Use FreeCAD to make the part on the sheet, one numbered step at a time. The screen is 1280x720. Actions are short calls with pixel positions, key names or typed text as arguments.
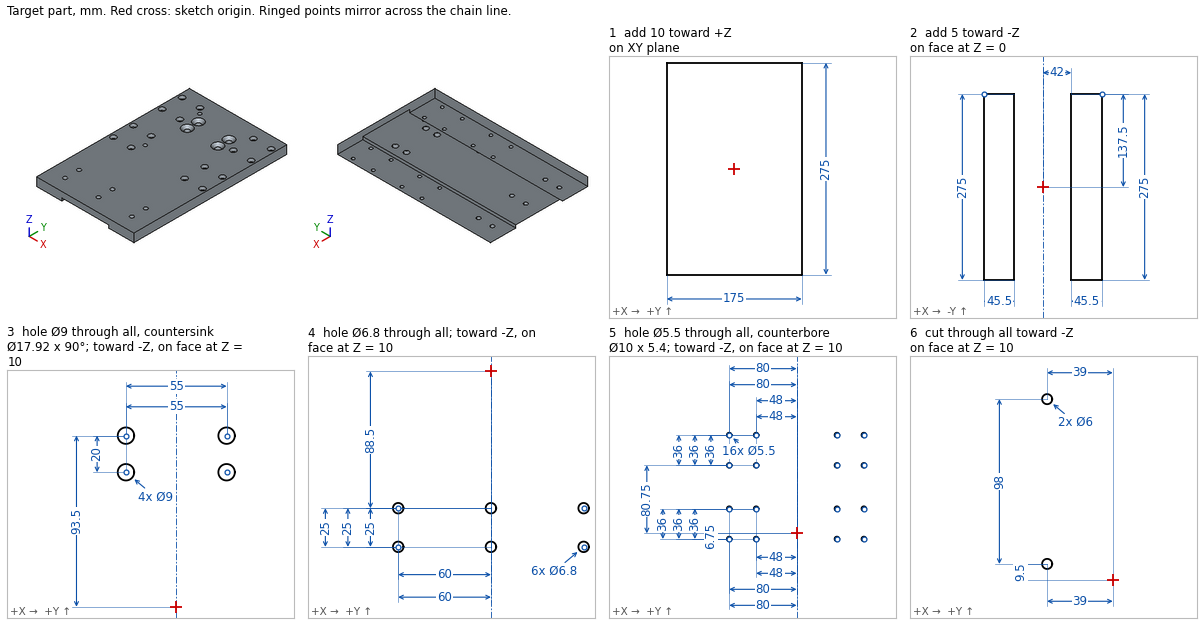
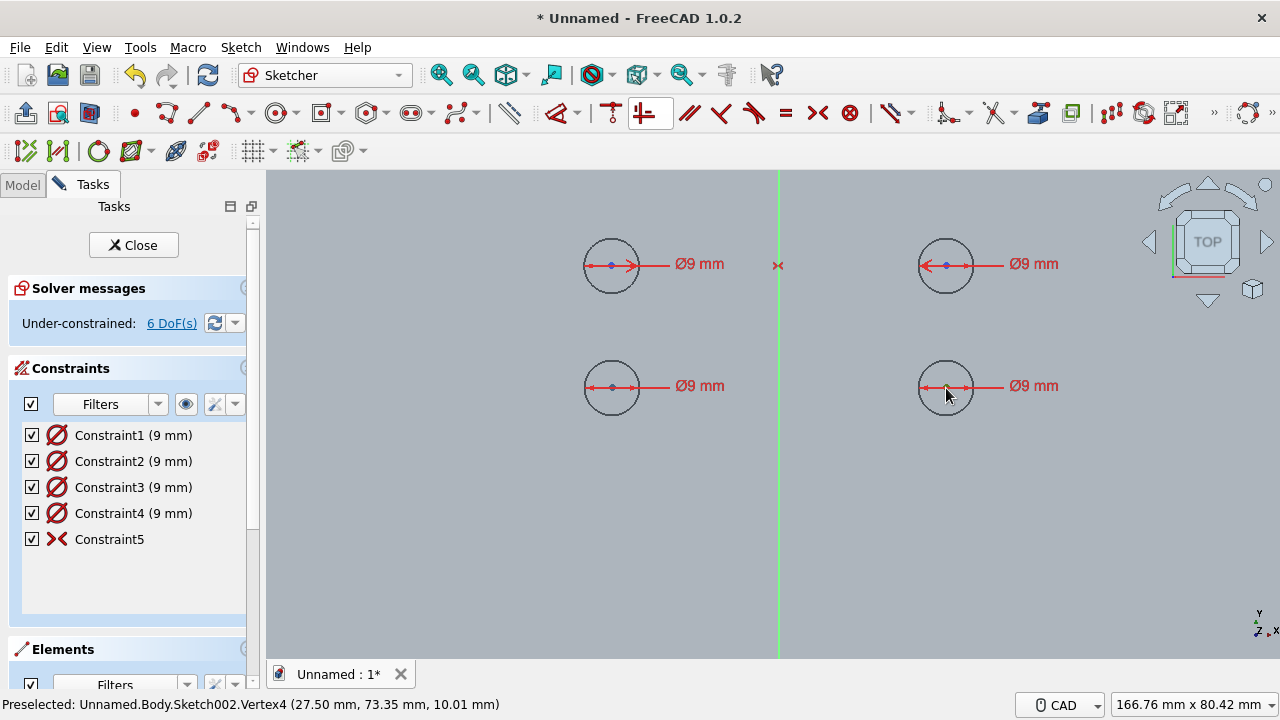
click(779, 600)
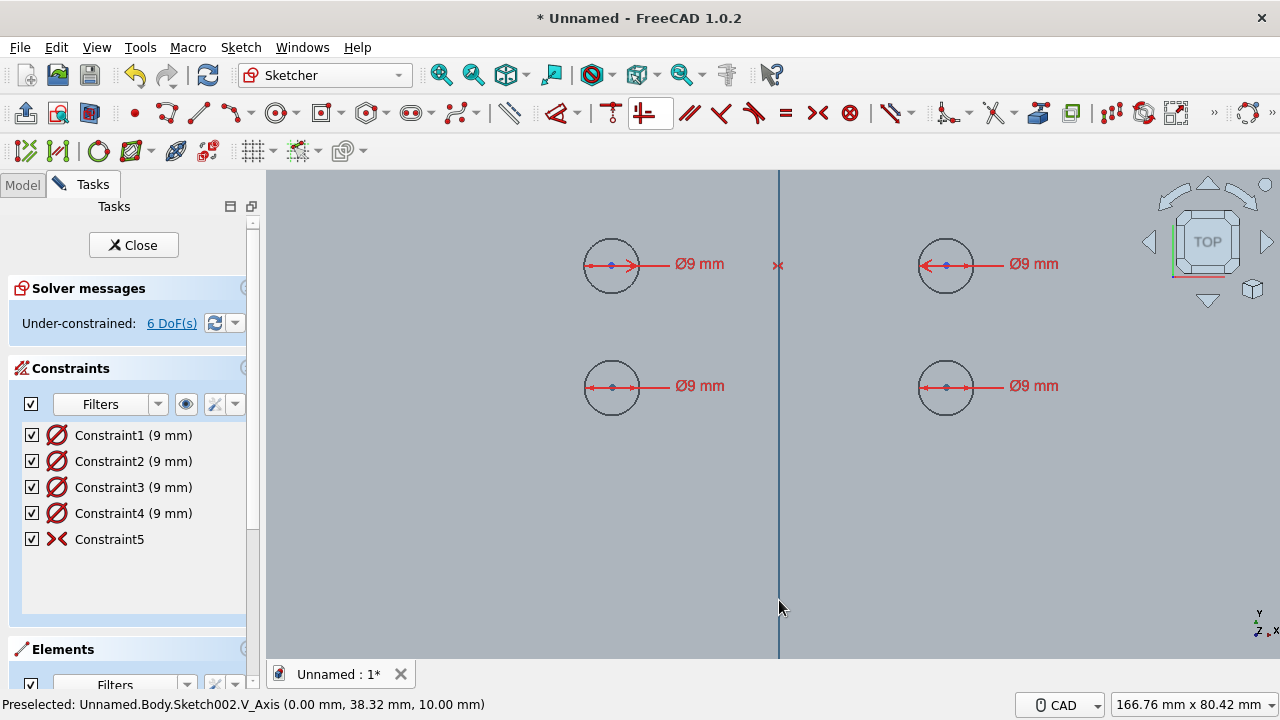
key(s)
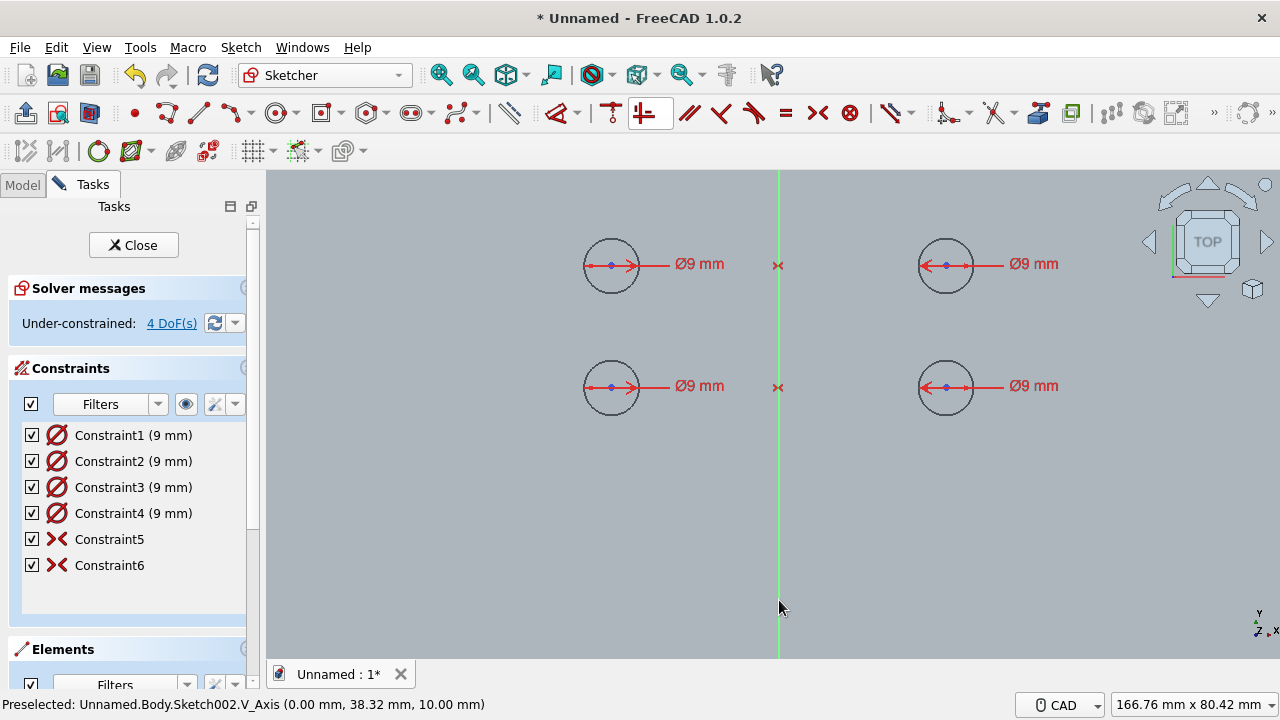
key(d)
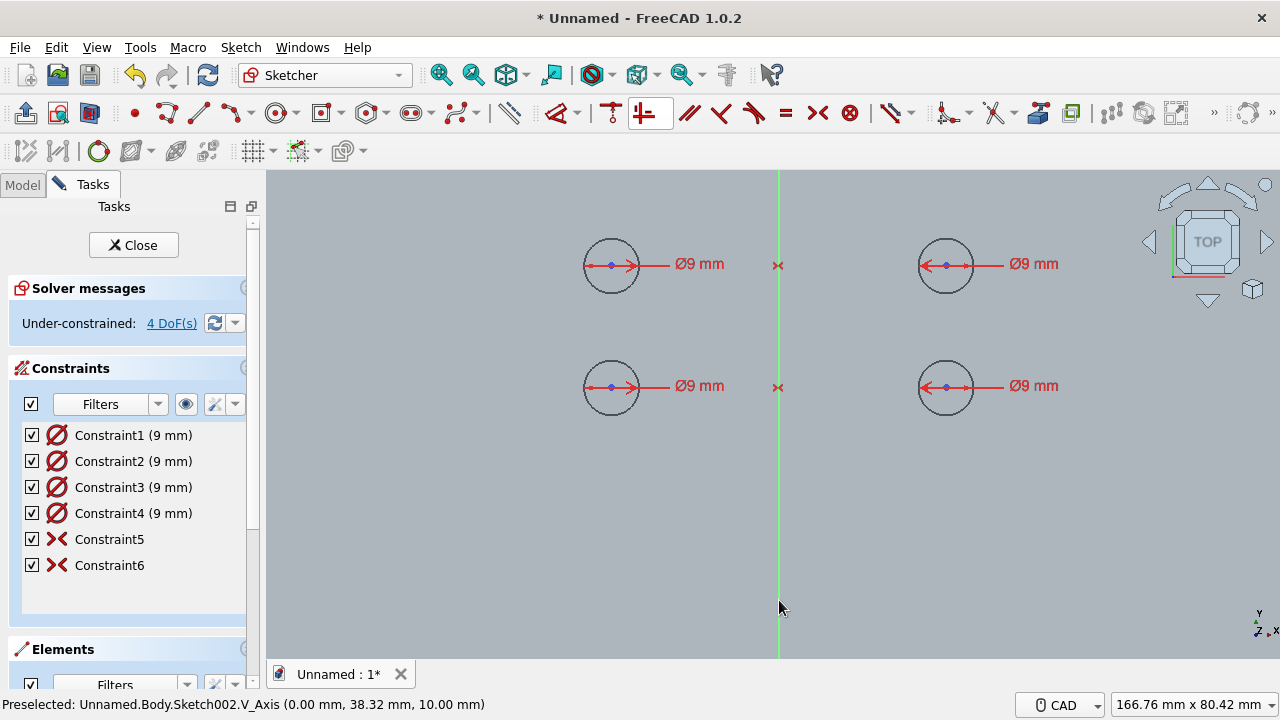
click(612, 266)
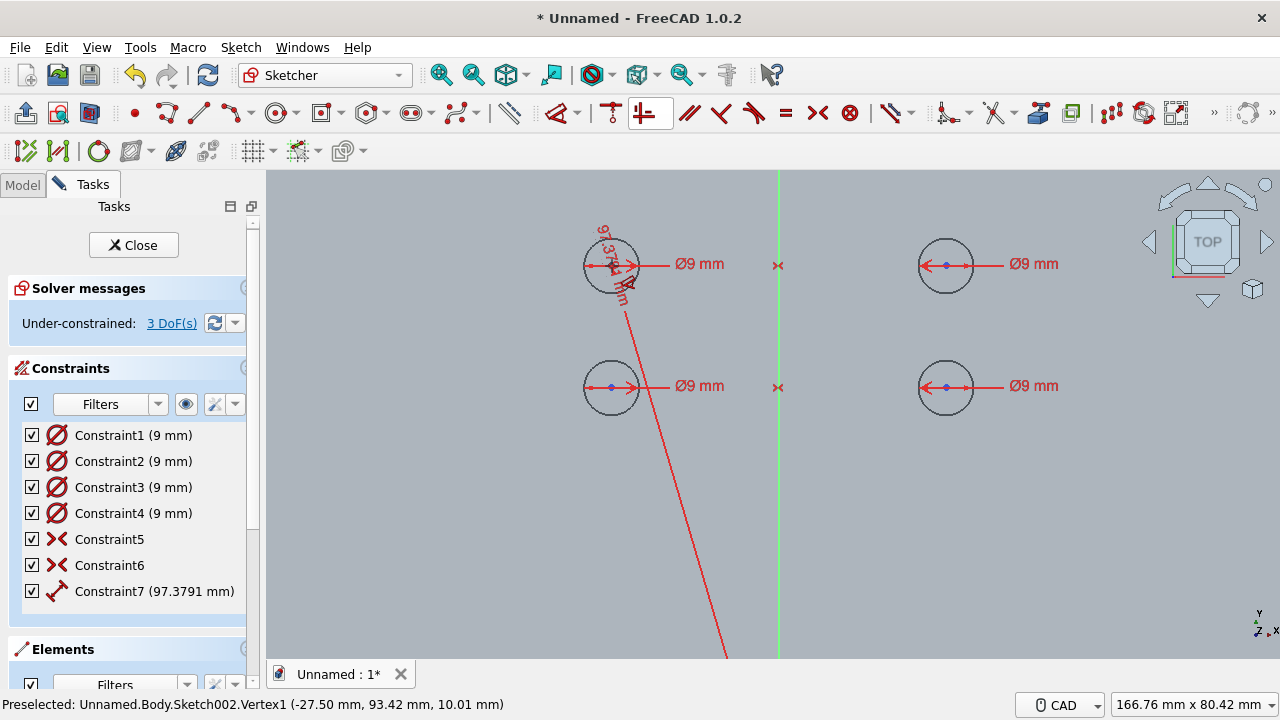
click(612, 388)
click(578, 327)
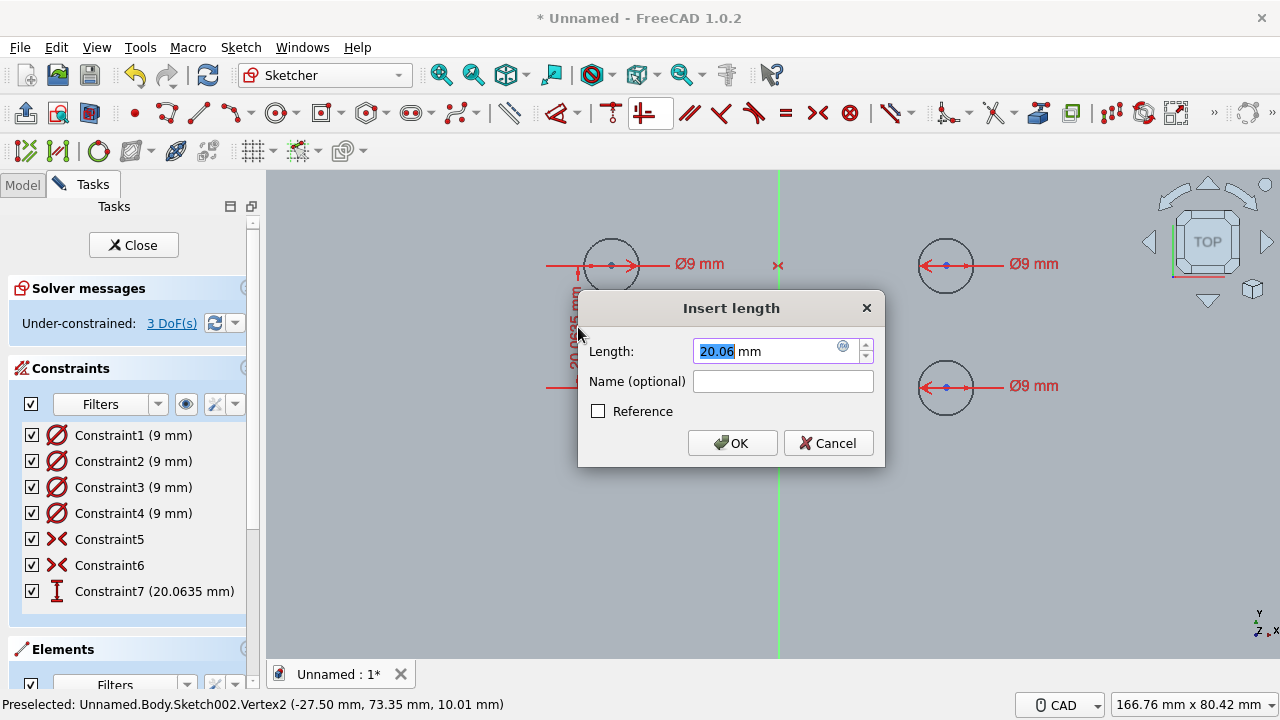
text(20)
key(Return)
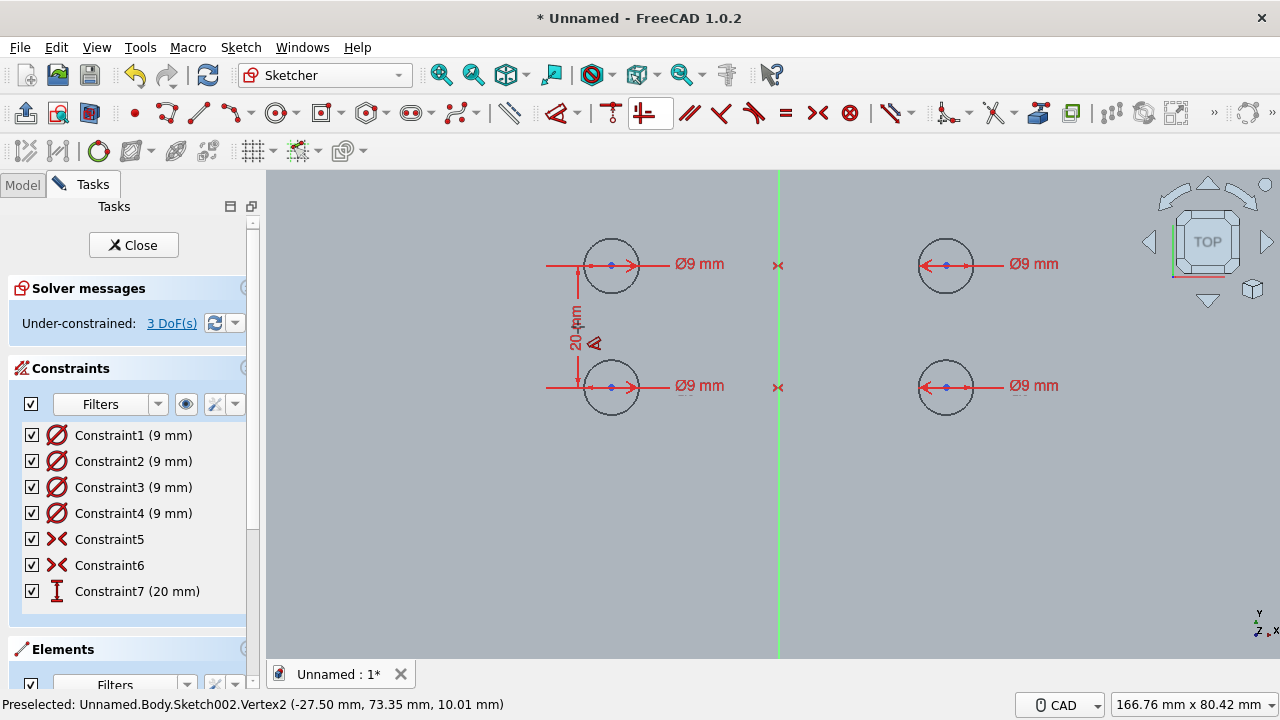
click(612, 266)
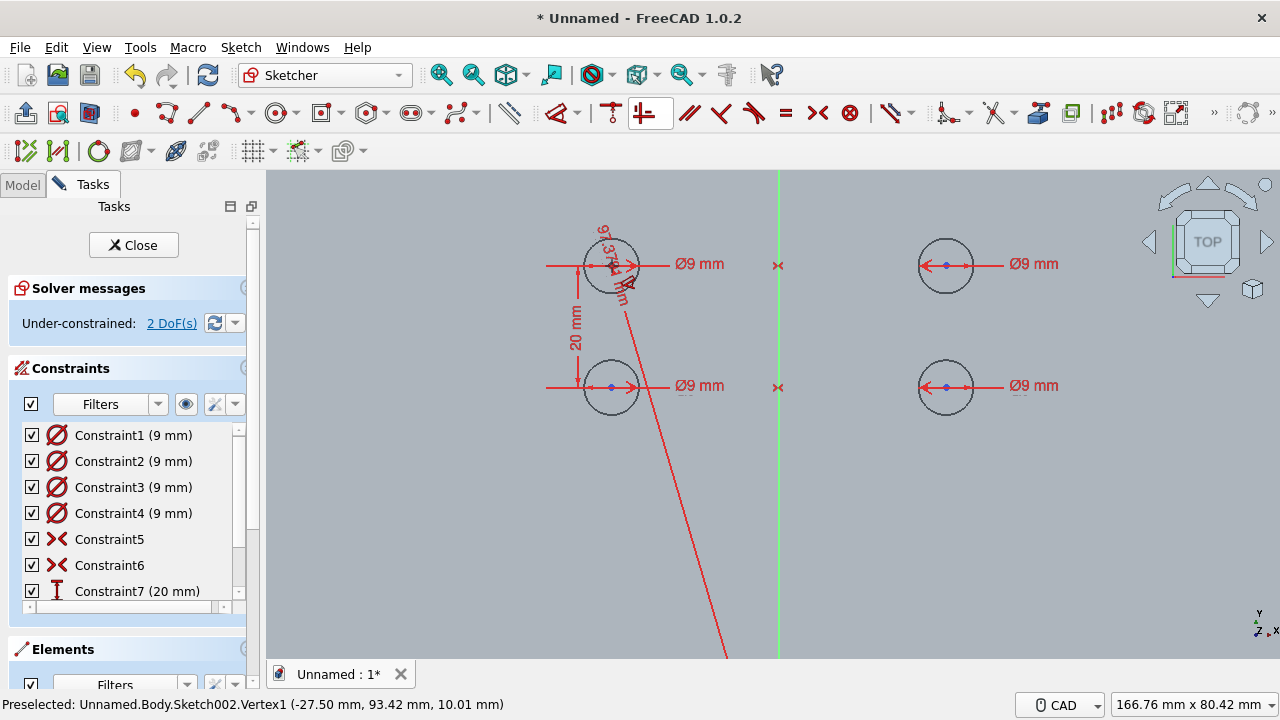
click(946, 266)
click(702, 232)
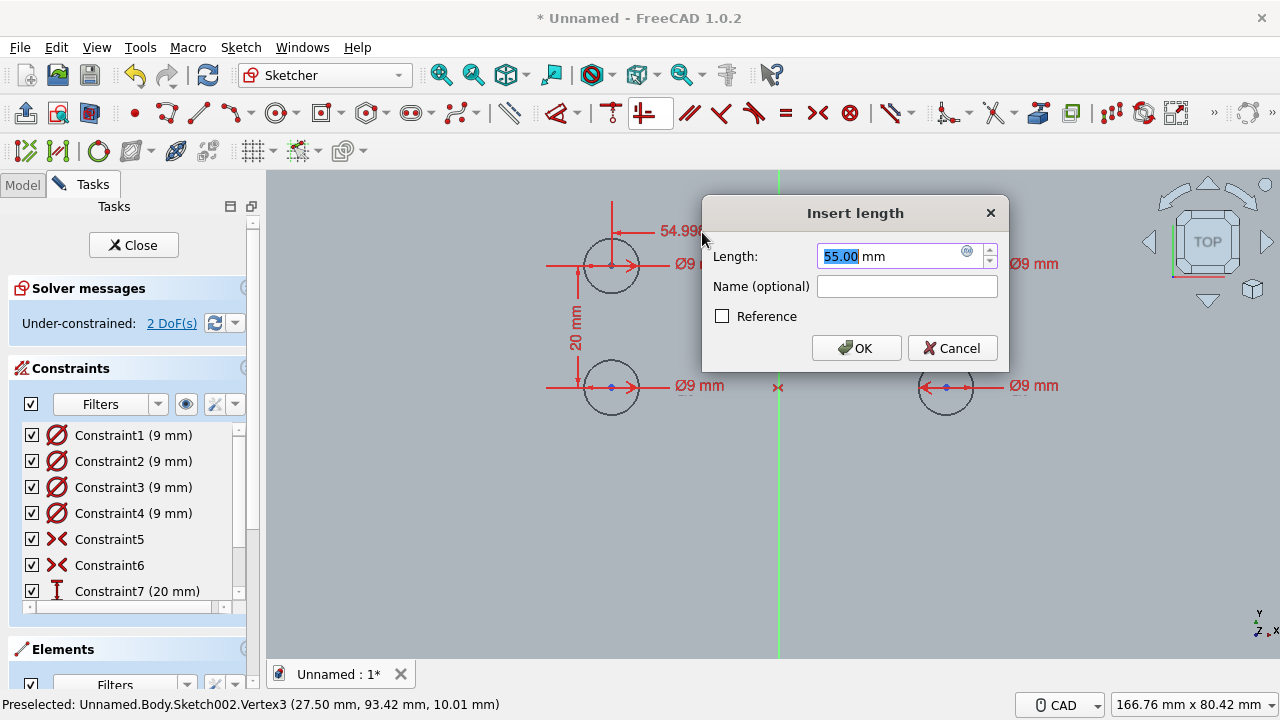
text(55)
key(Return)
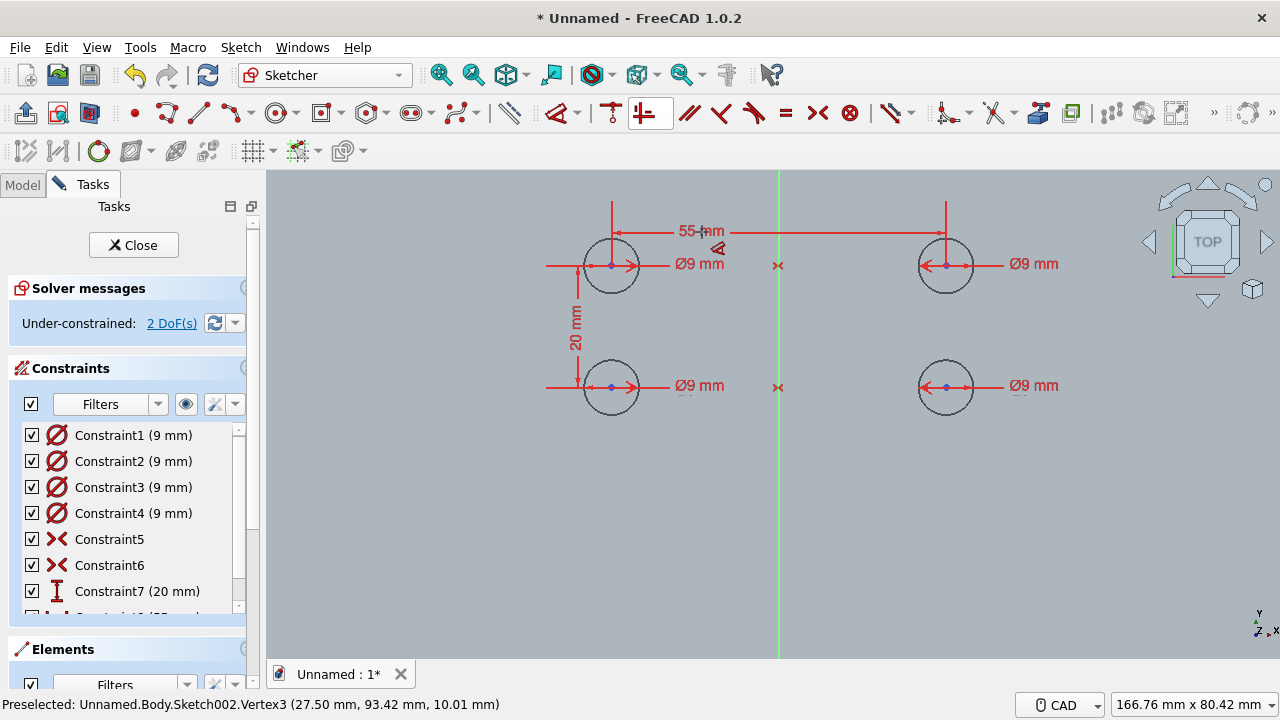
click(612, 388)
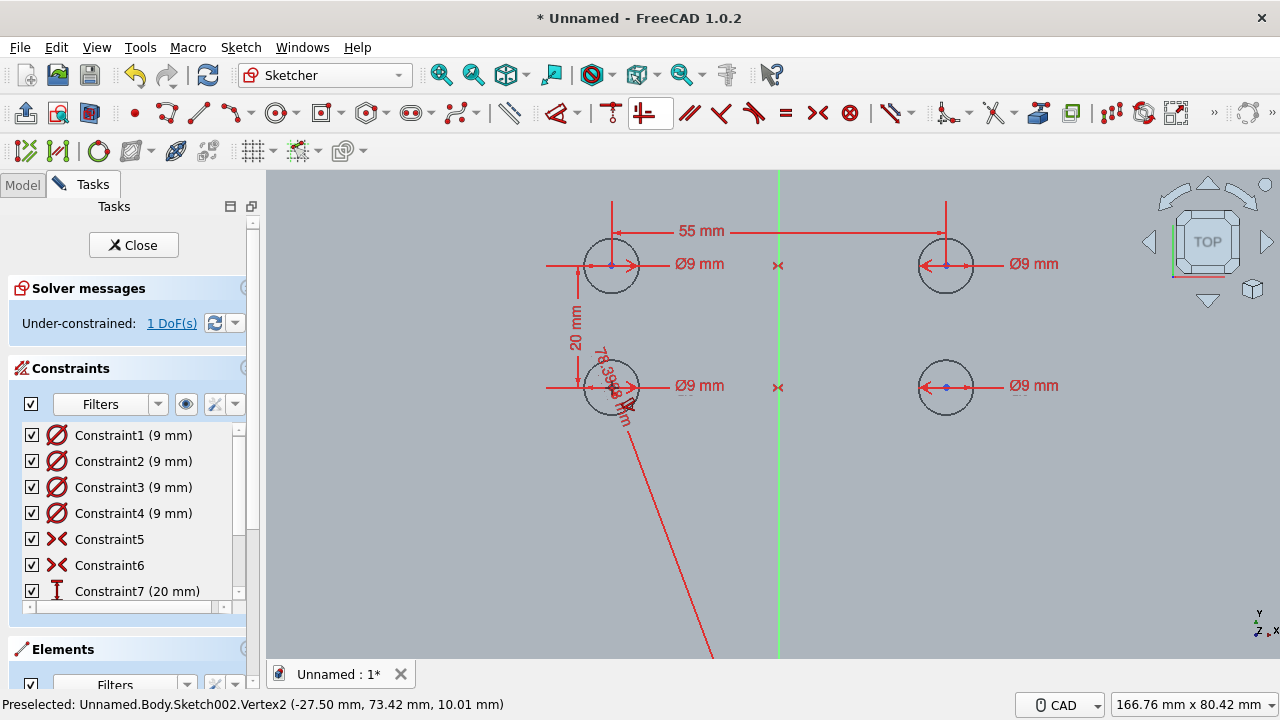
click(946, 266)
click(856, 232)